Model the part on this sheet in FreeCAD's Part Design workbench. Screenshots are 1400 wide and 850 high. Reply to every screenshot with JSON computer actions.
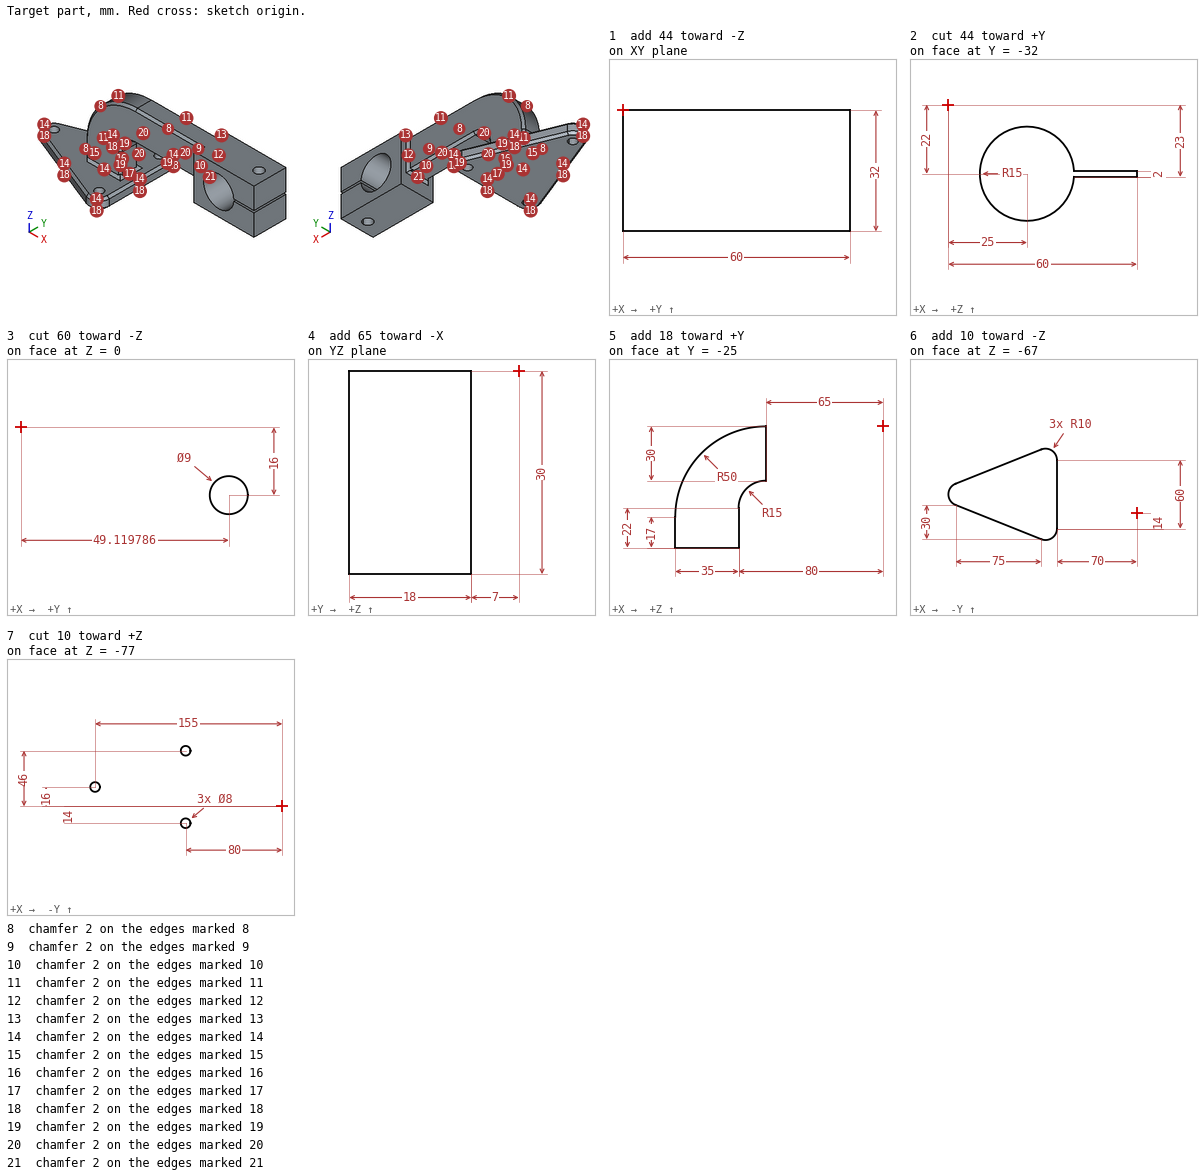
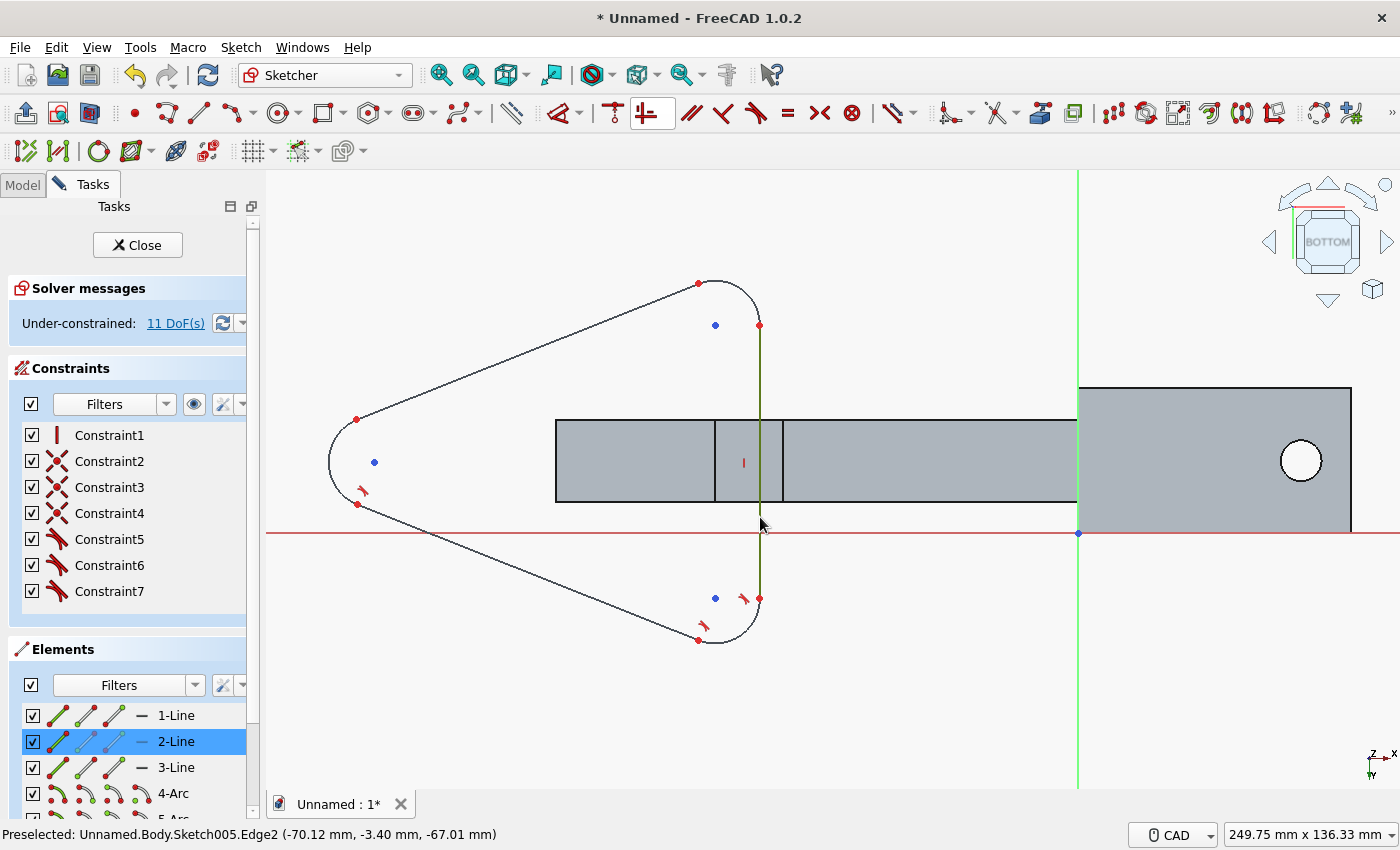
{"action": "left_click", "coordinate": [753, 301]}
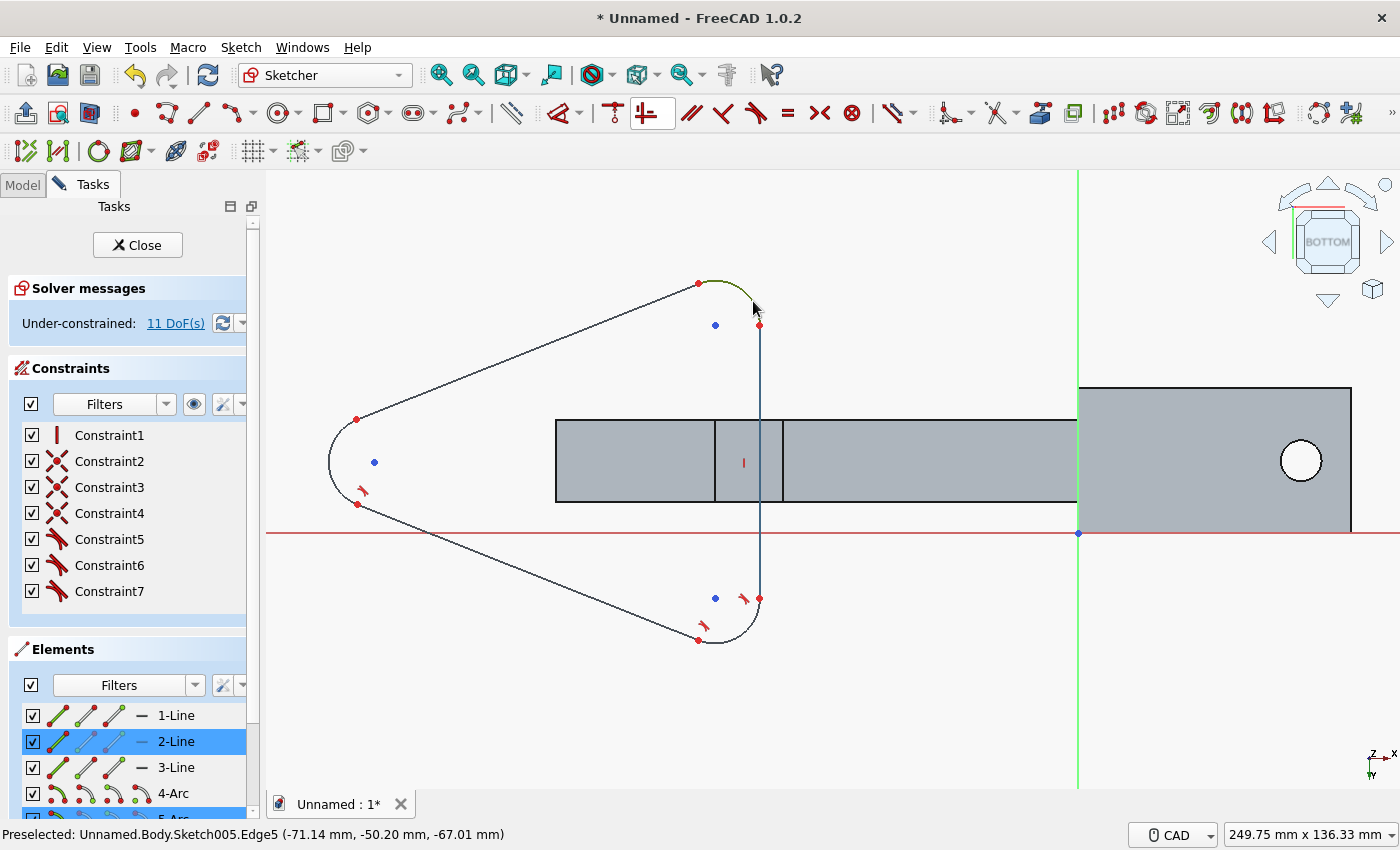
{"action": "left_click", "coordinate": [756, 114]}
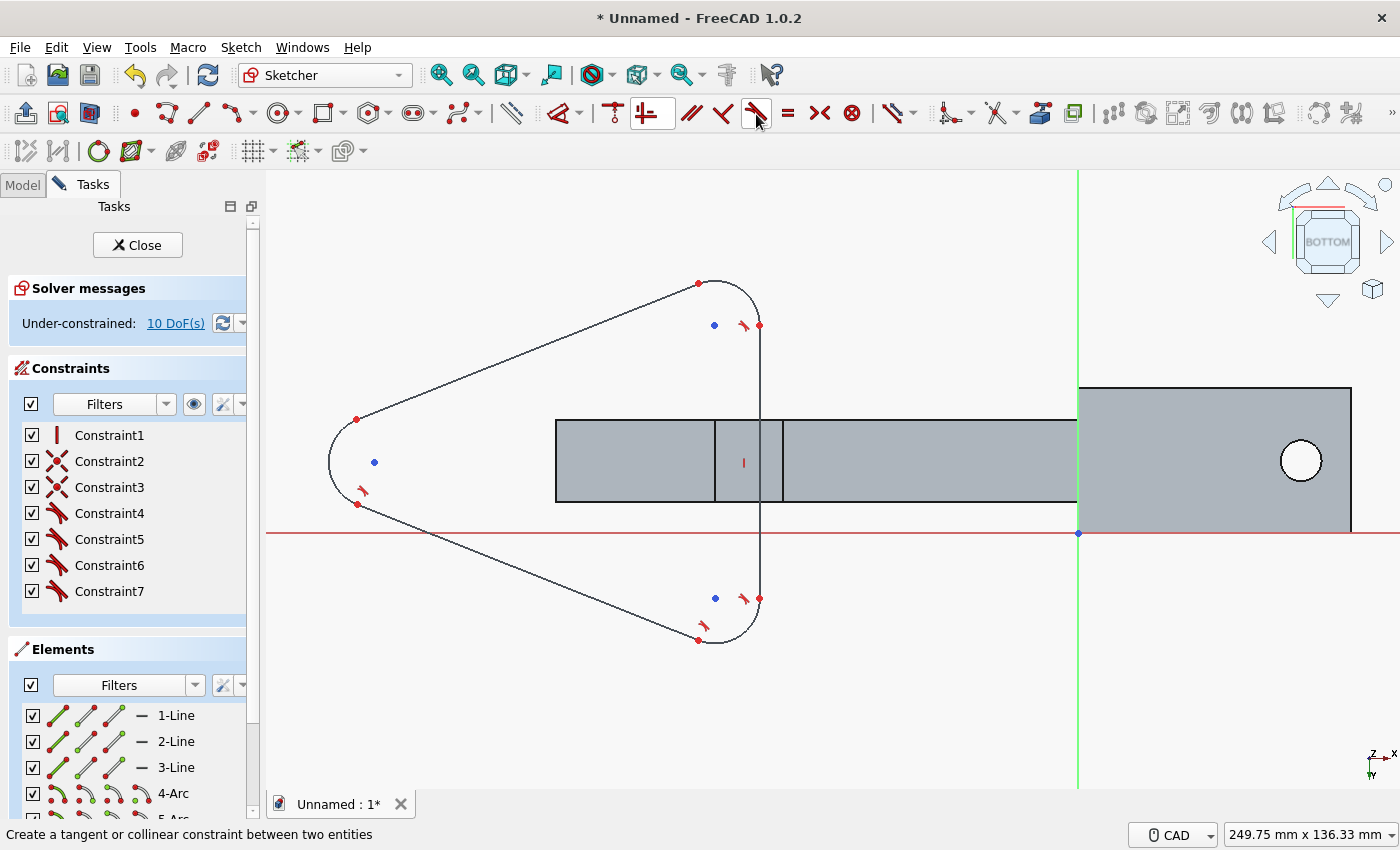
{"action": "left_click", "coordinate": [596, 325]}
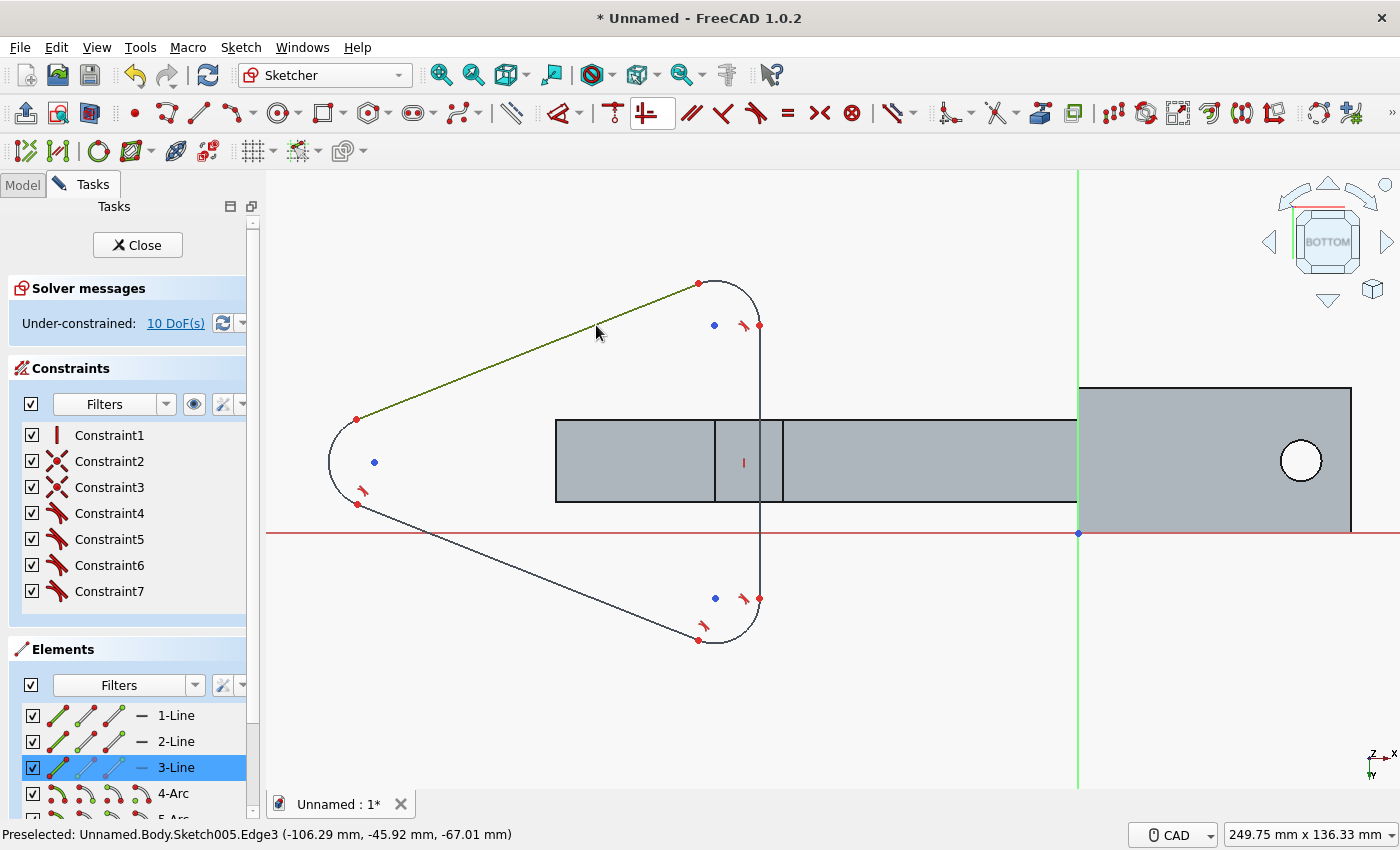
{"action": "left_click", "coordinate": [752, 301]}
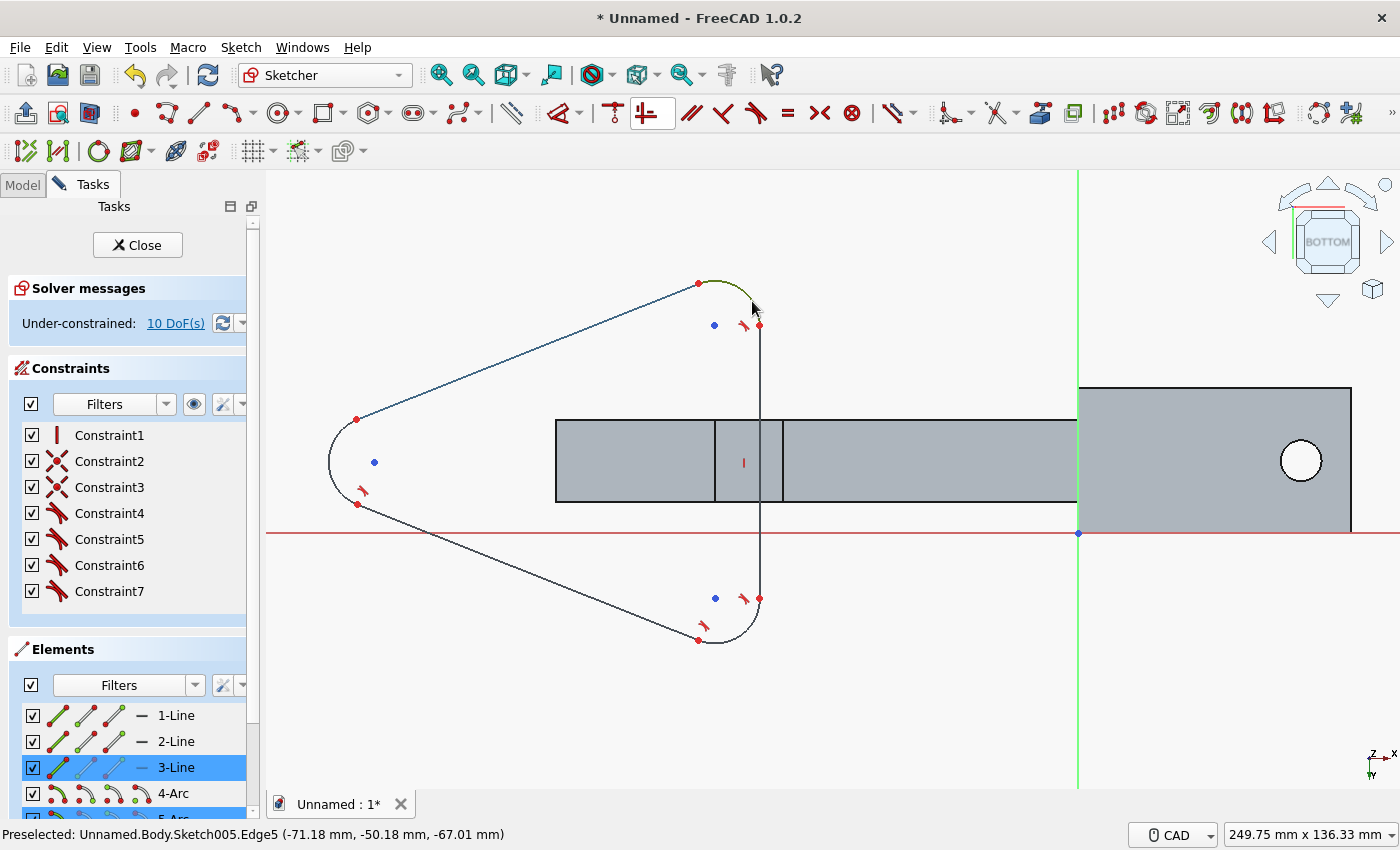
{"action": "left_click", "coordinate": [756, 114]}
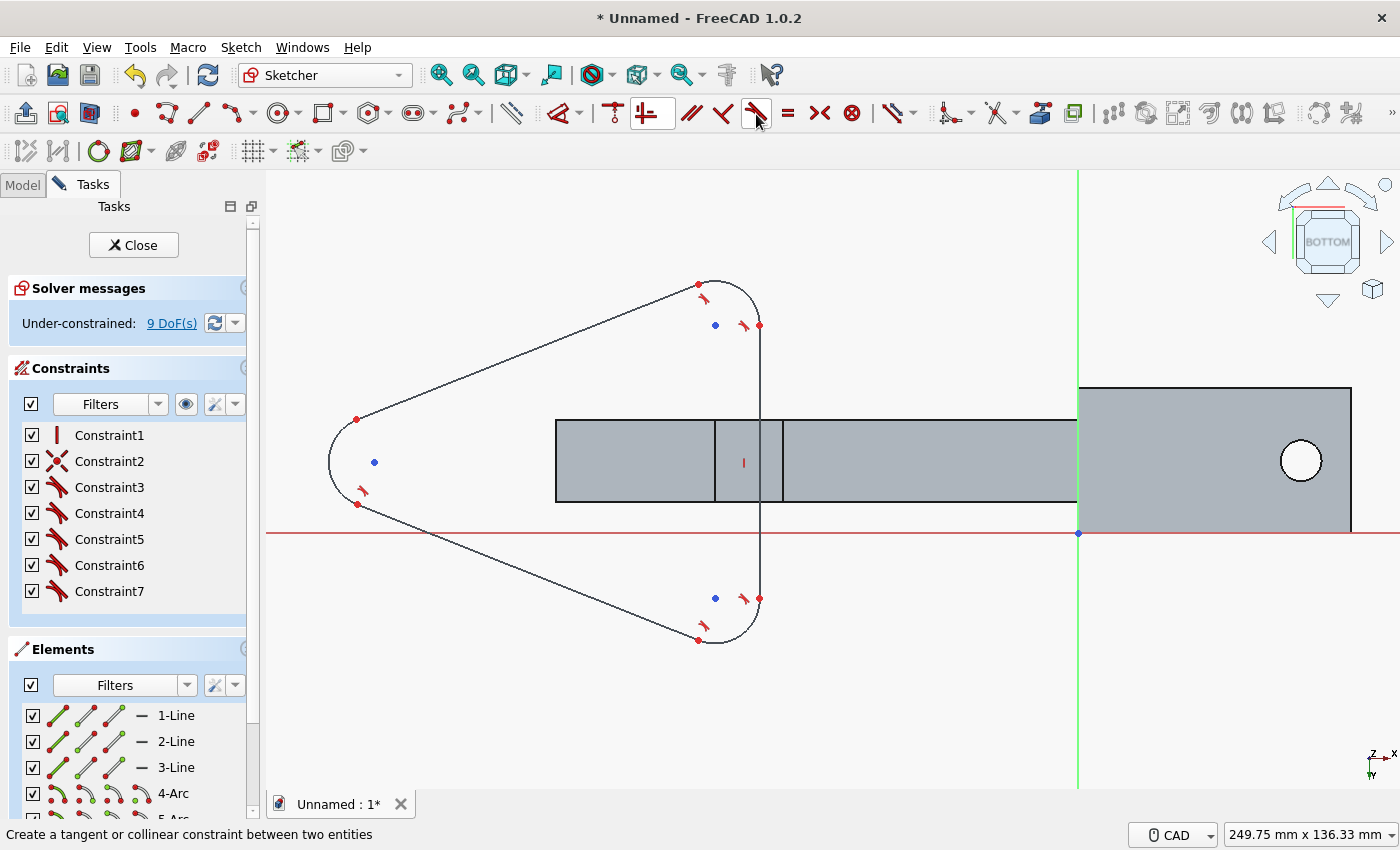
{"action": "left_click", "coordinate": [596, 325]}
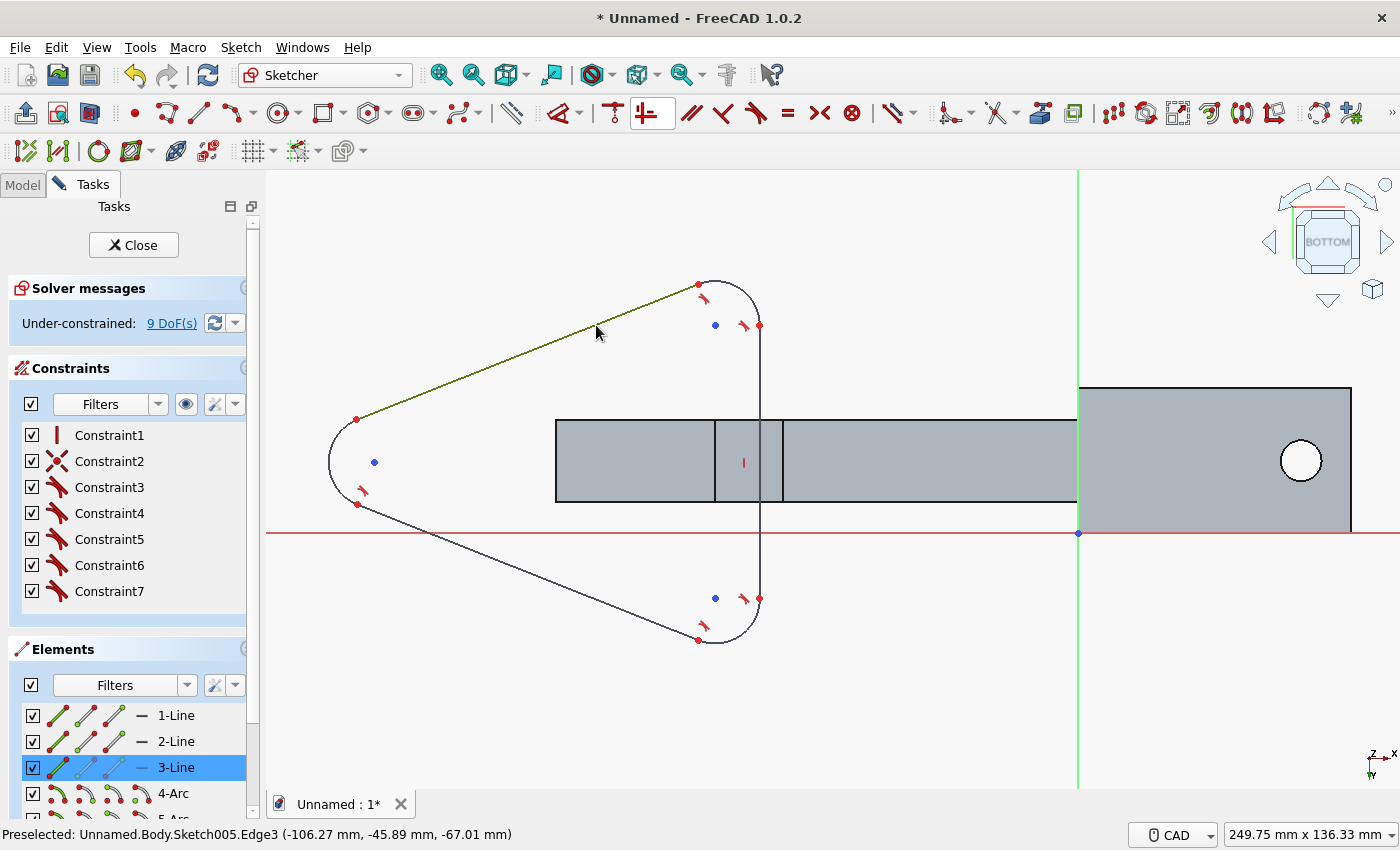
{"action": "left_click", "coordinate": [334, 442]}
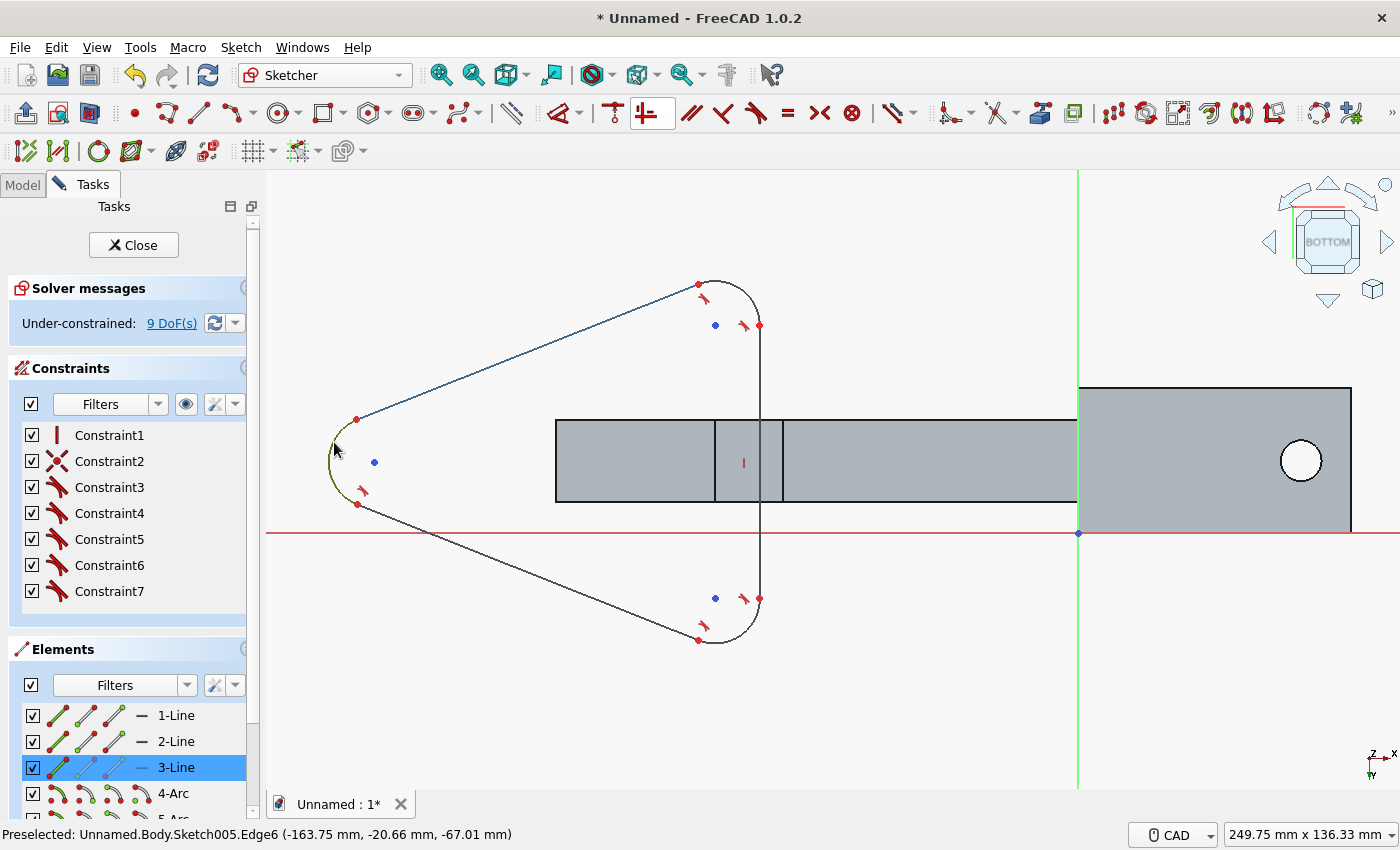
{"action": "left_click", "coordinate": [756, 114]}